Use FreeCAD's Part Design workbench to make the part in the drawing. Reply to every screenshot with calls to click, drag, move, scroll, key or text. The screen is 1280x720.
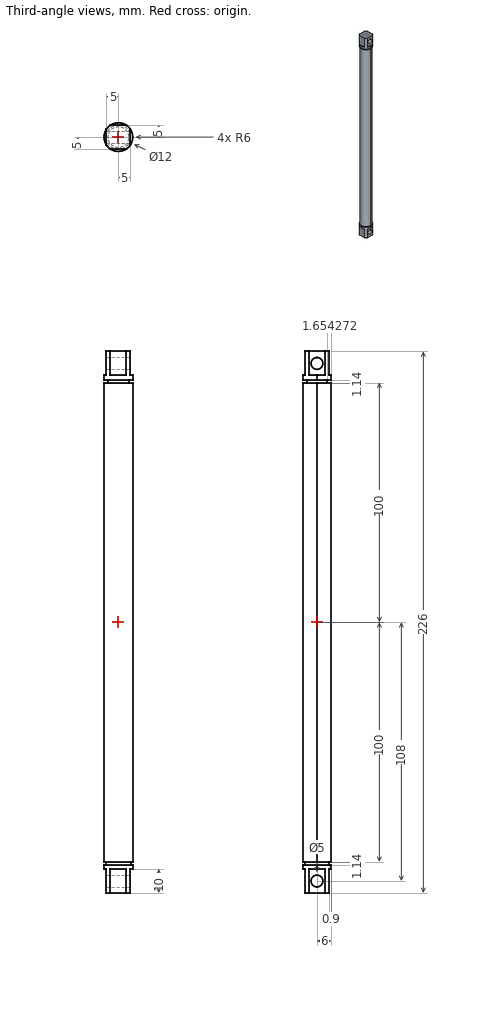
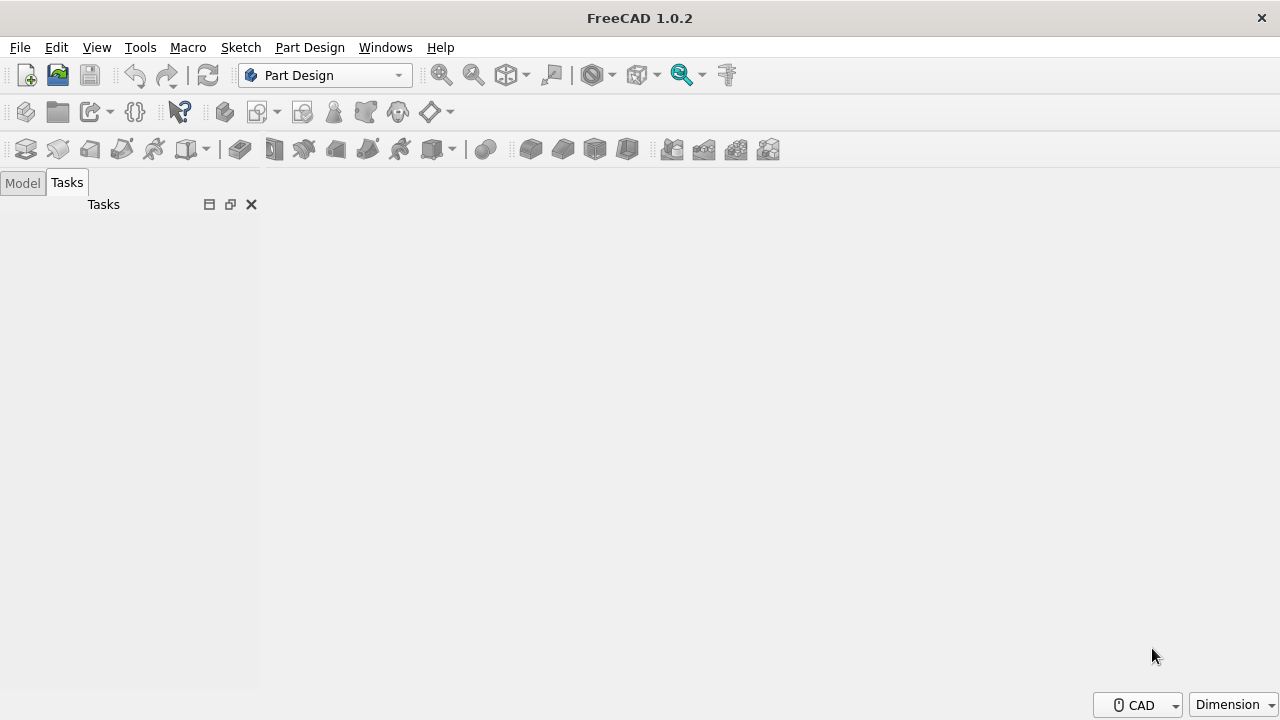
click(26, 76)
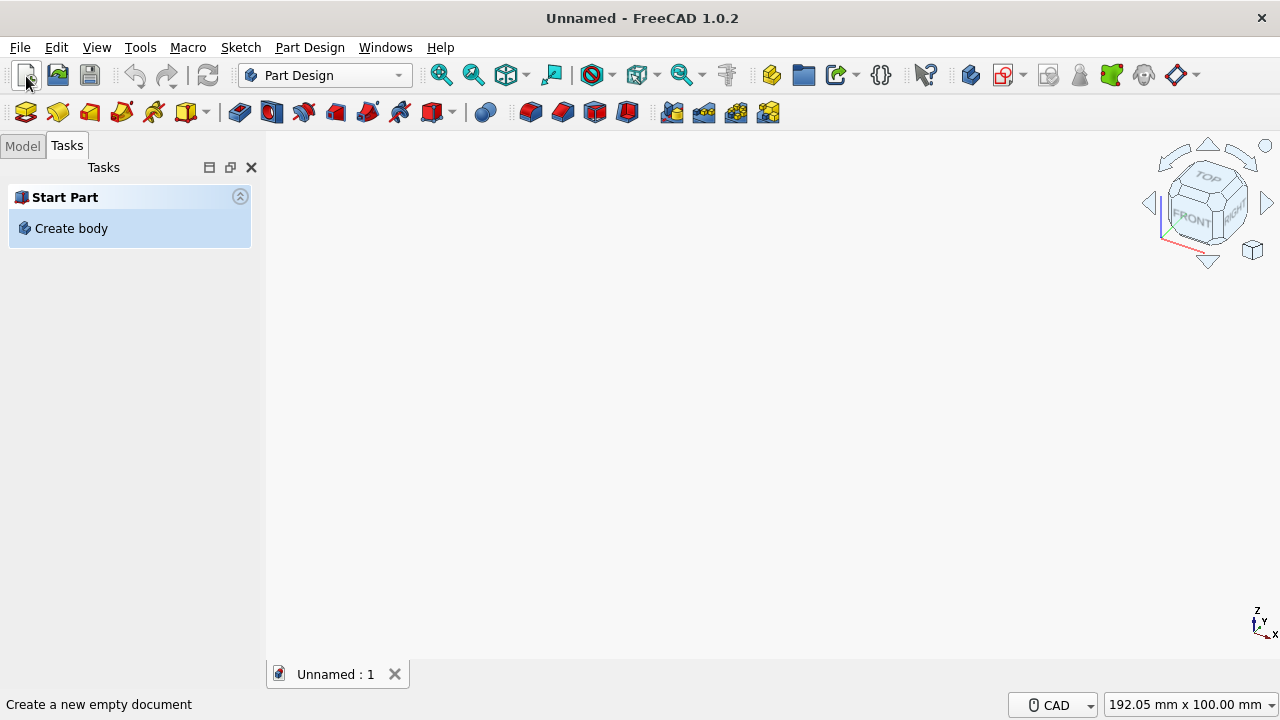
click(1004, 76)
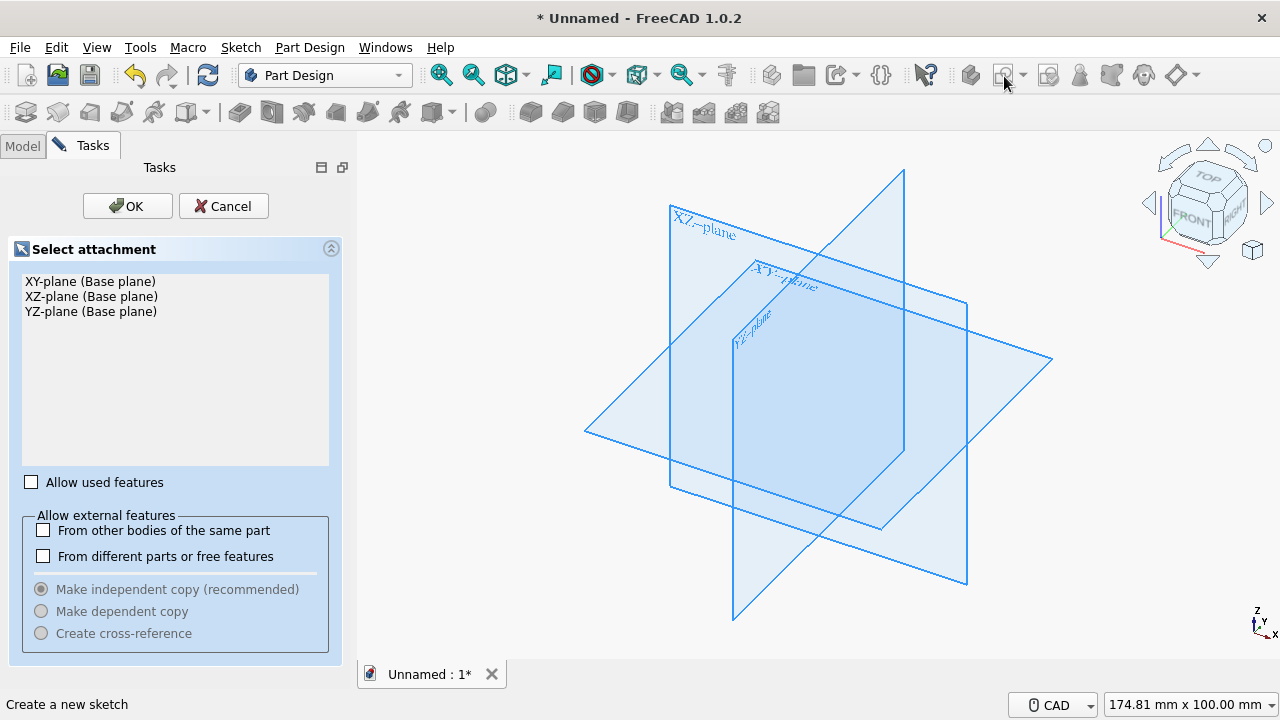
click(82, 282)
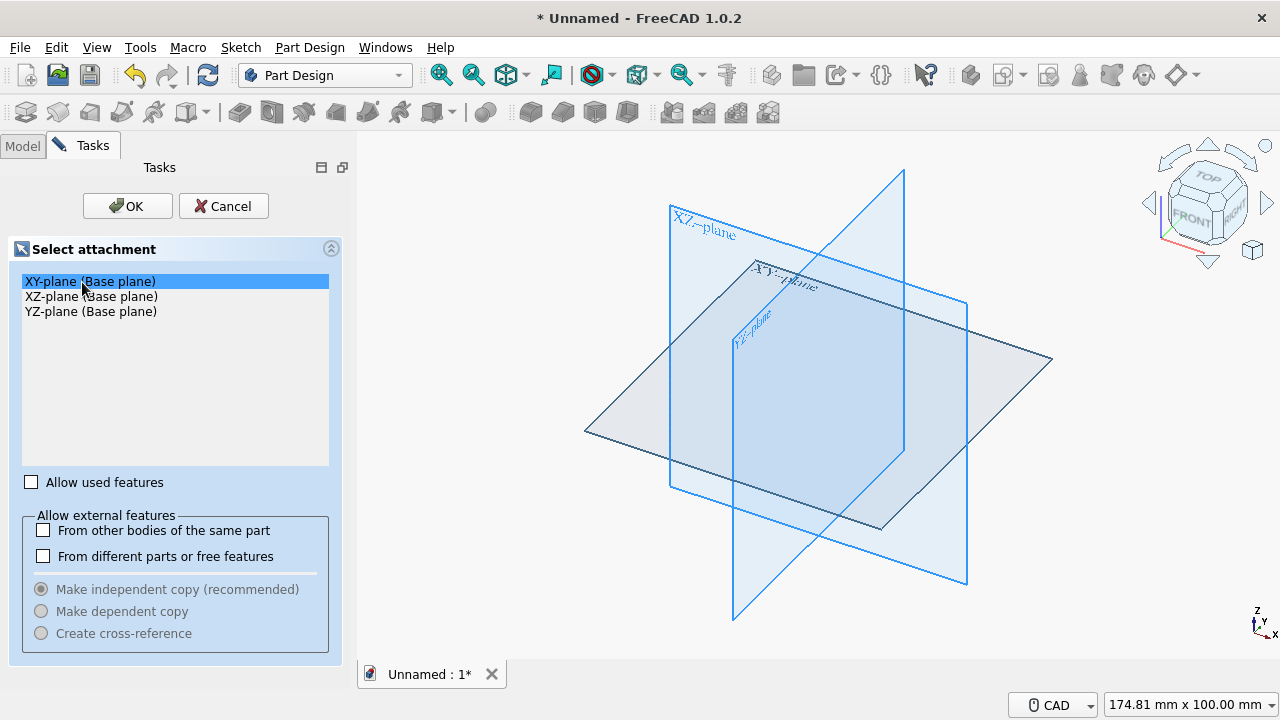
click(128, 206)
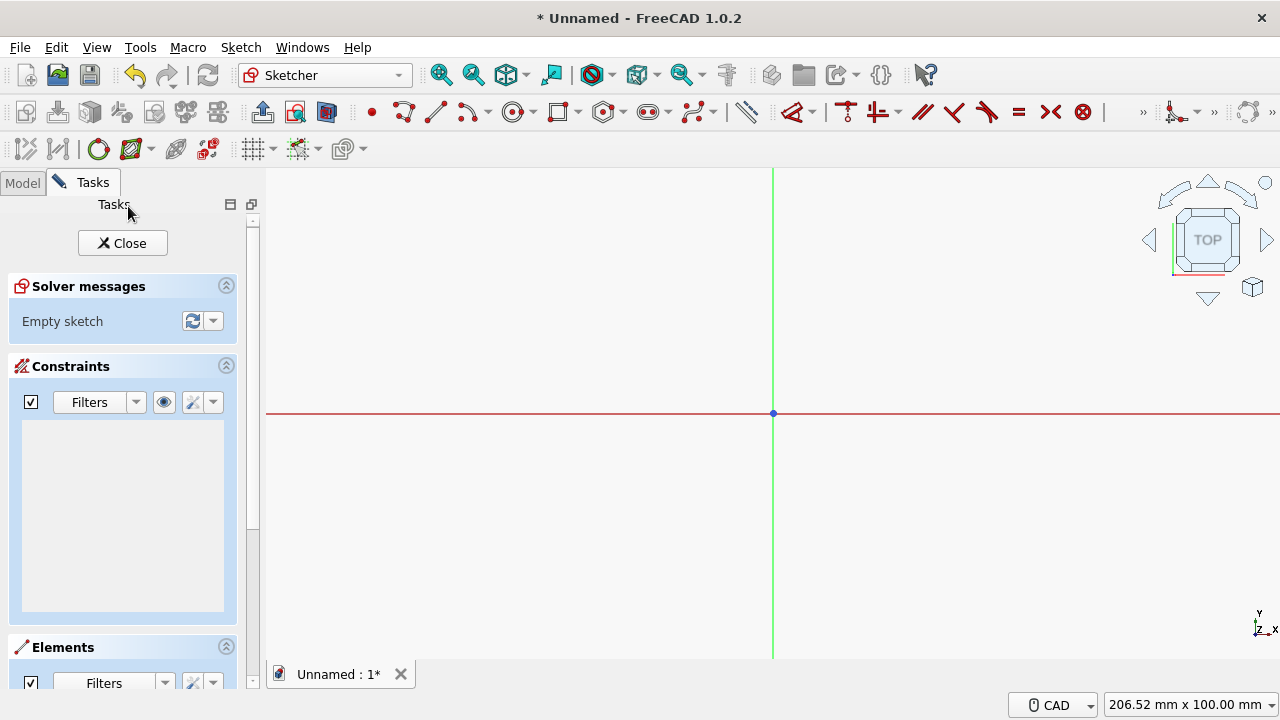
scroll(790, 414, up, 8)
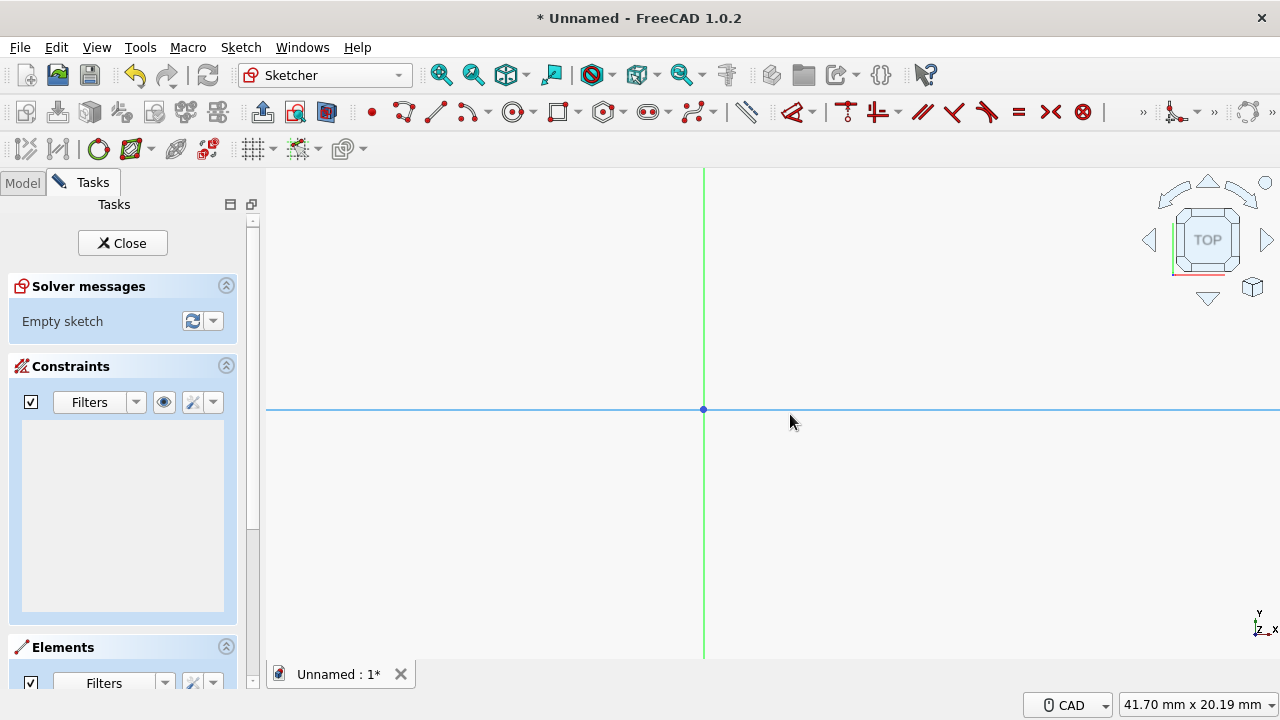
key(g)
key(c)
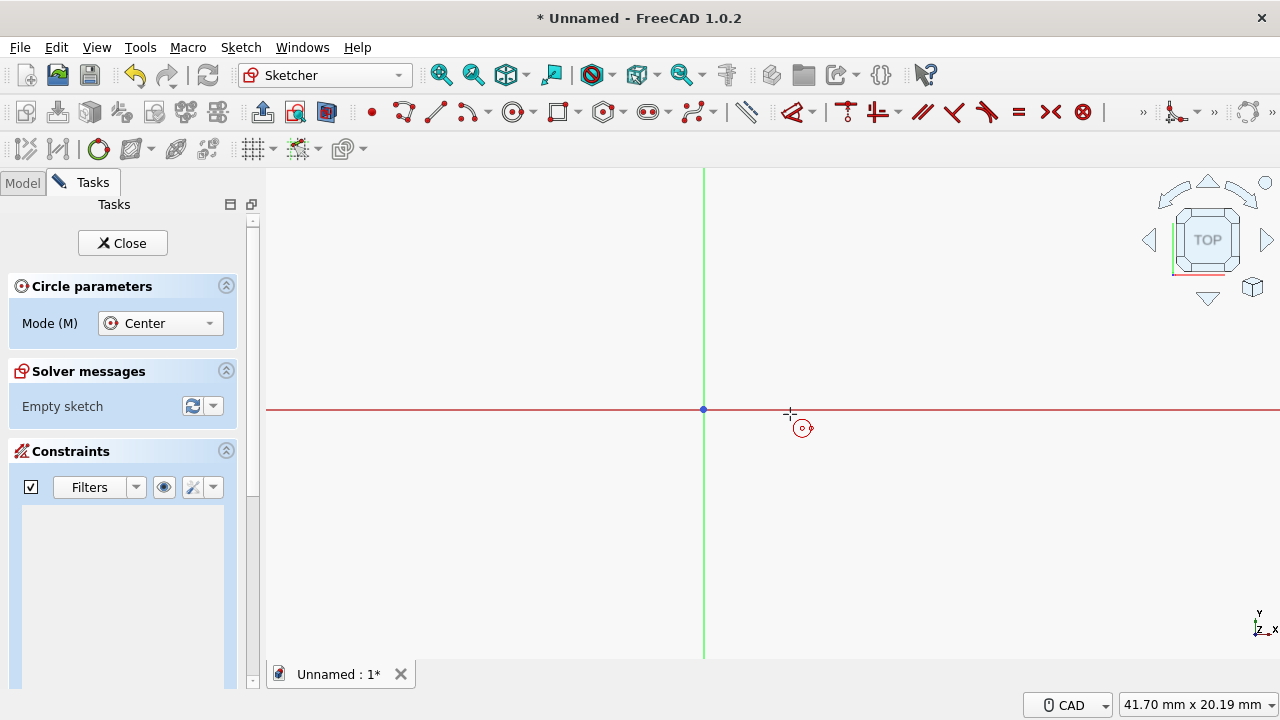
click(704, 410)
move(807, 306)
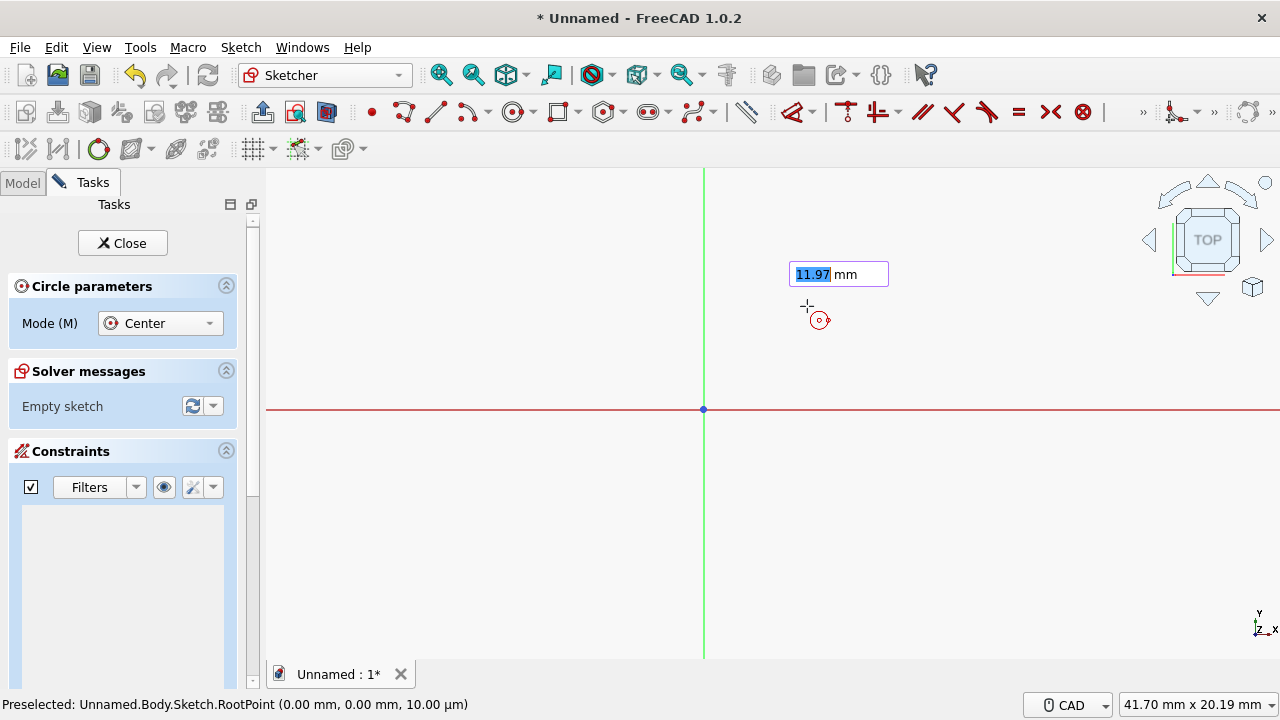
text(12)
key(Return)
key(Escape)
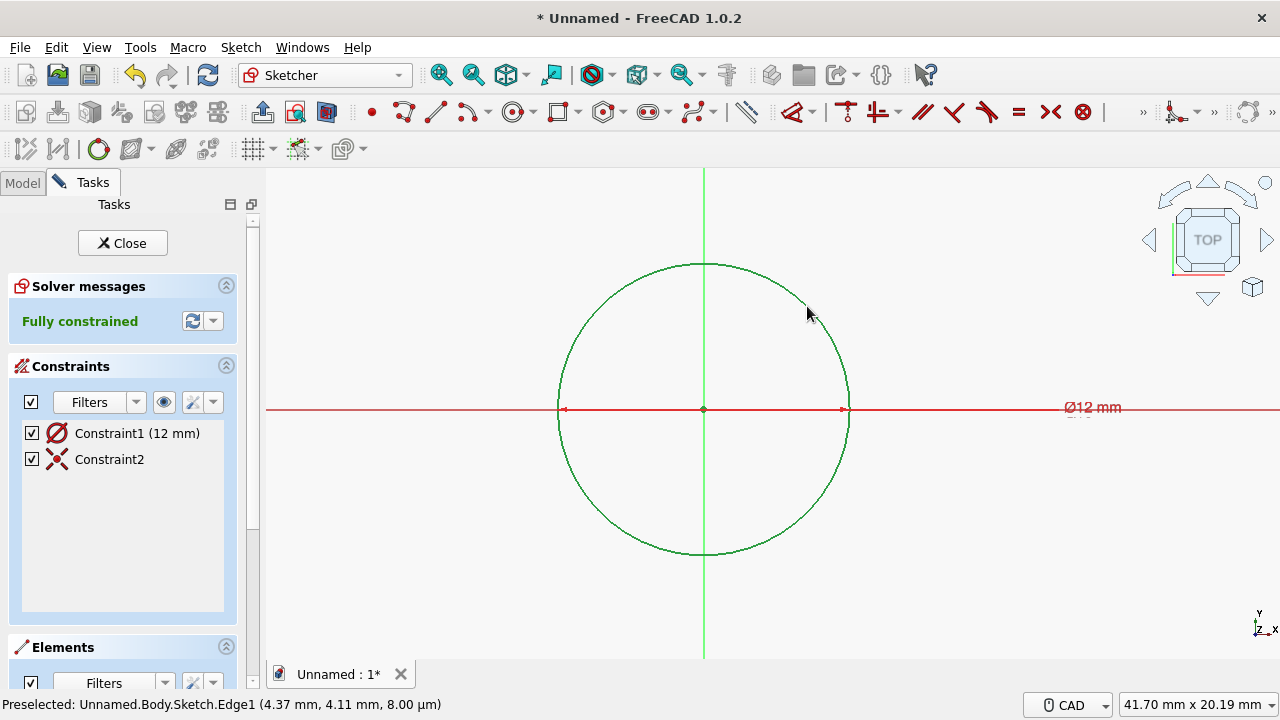
click(123, 243)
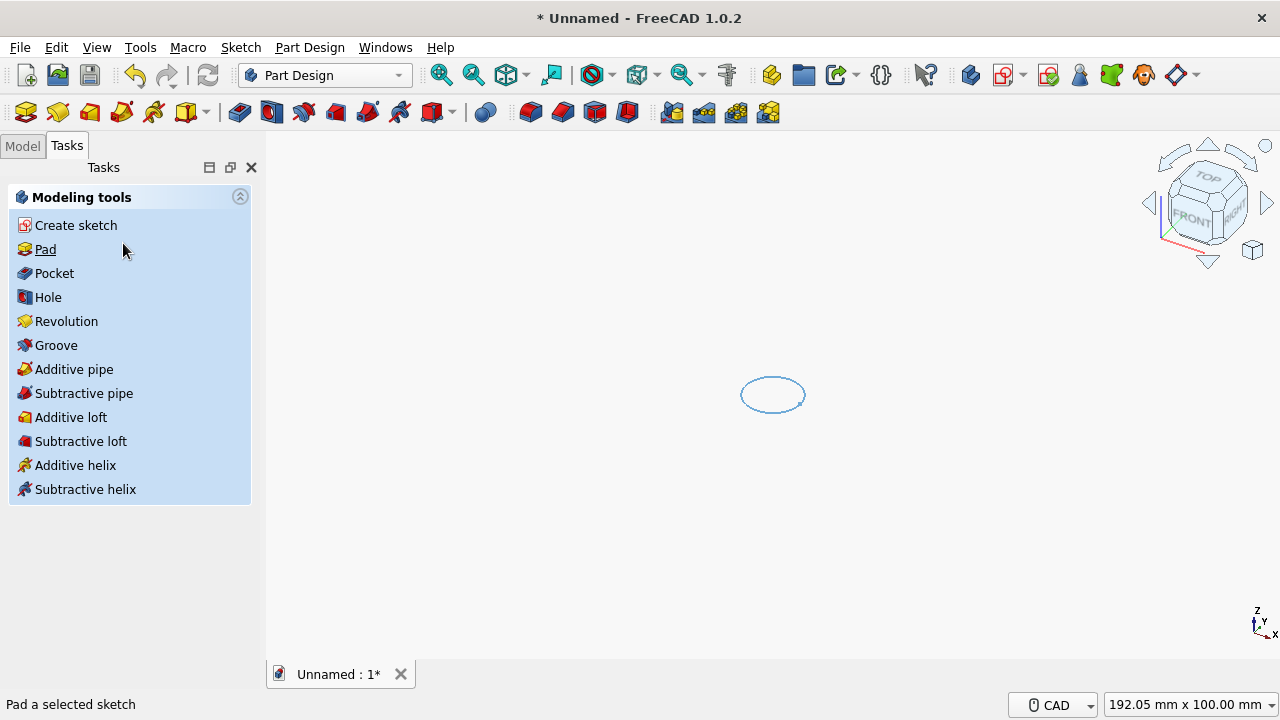
click(26, 112)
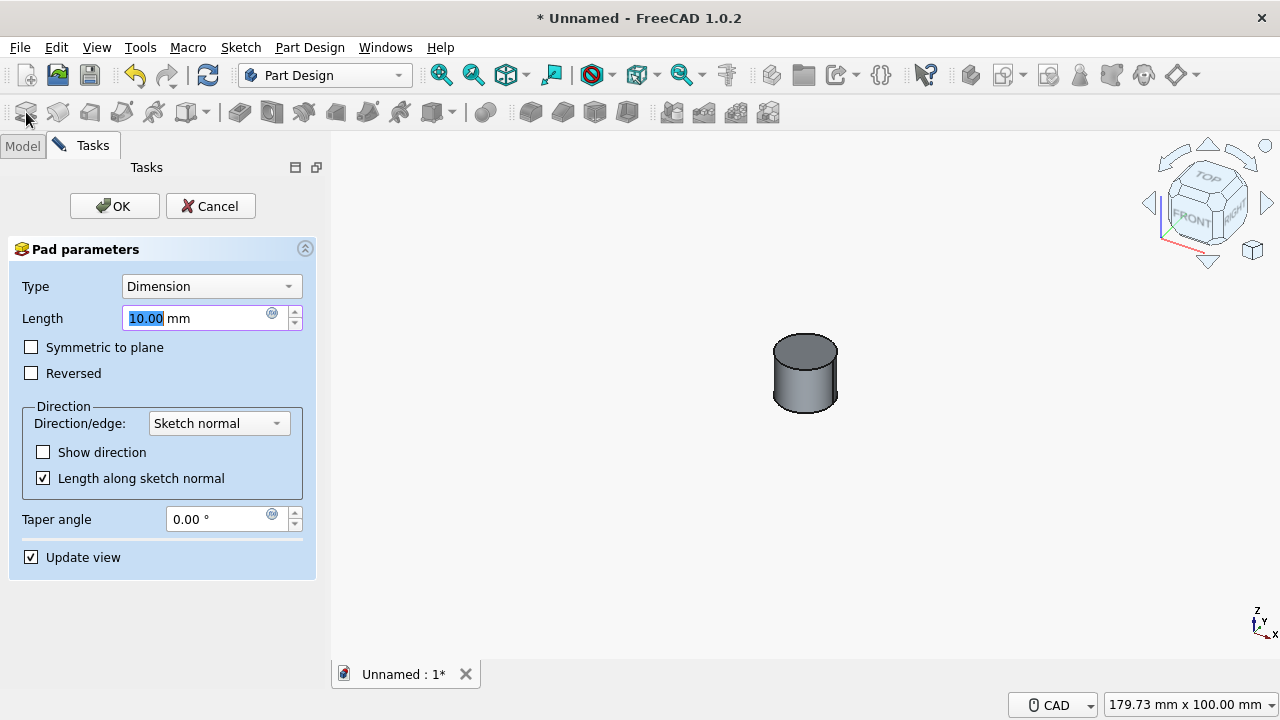
text(226)
key(Tab)